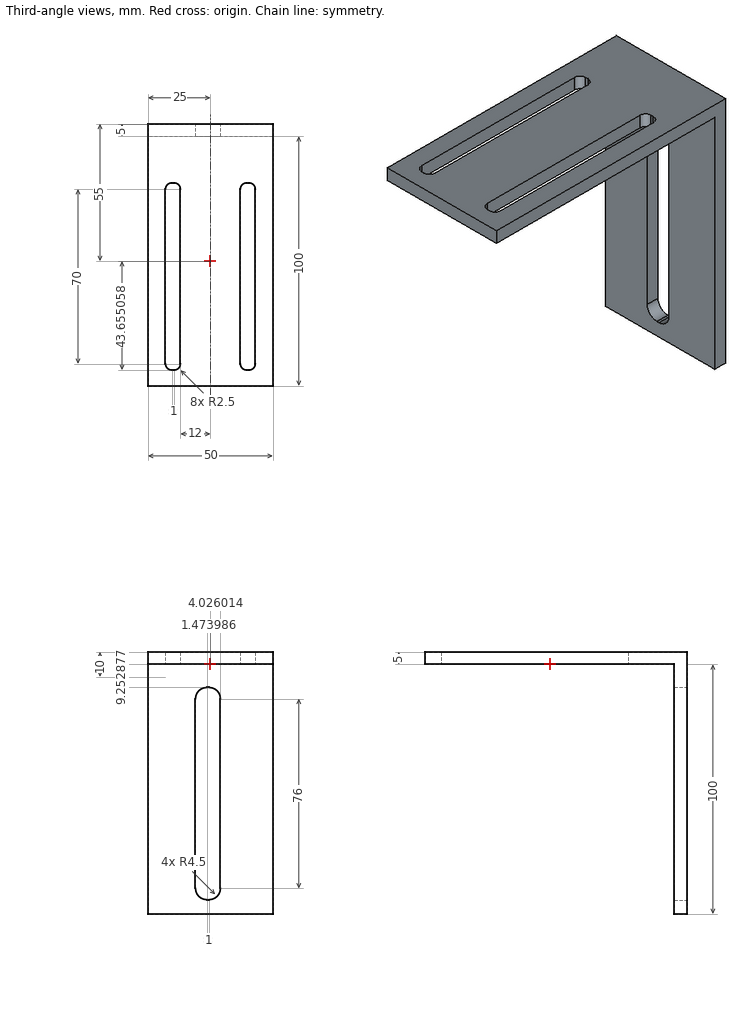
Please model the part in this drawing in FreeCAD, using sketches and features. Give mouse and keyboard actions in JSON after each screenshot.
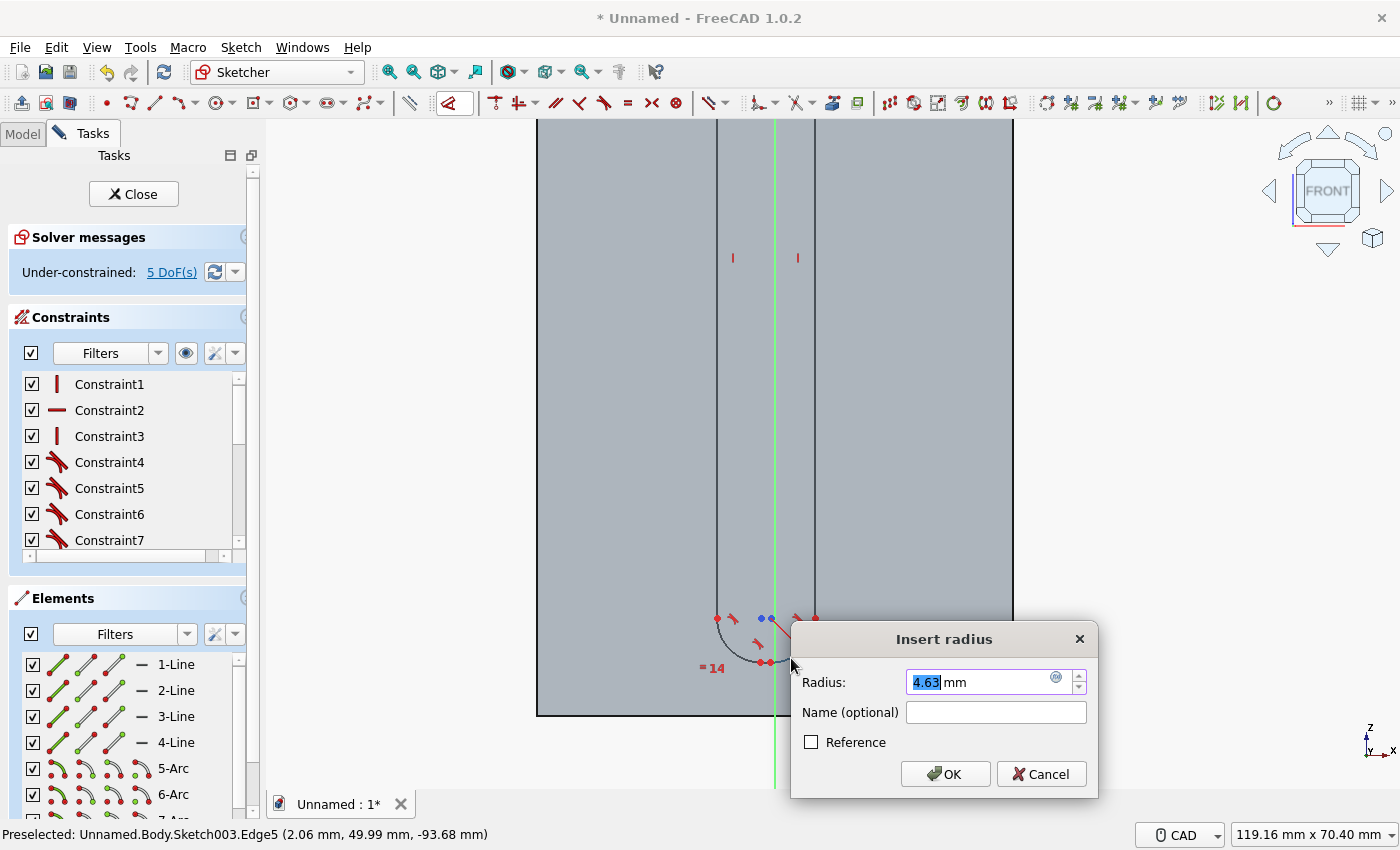
{"action": "type", "text": "4.5"}
{"action": "key", "text": "Return"}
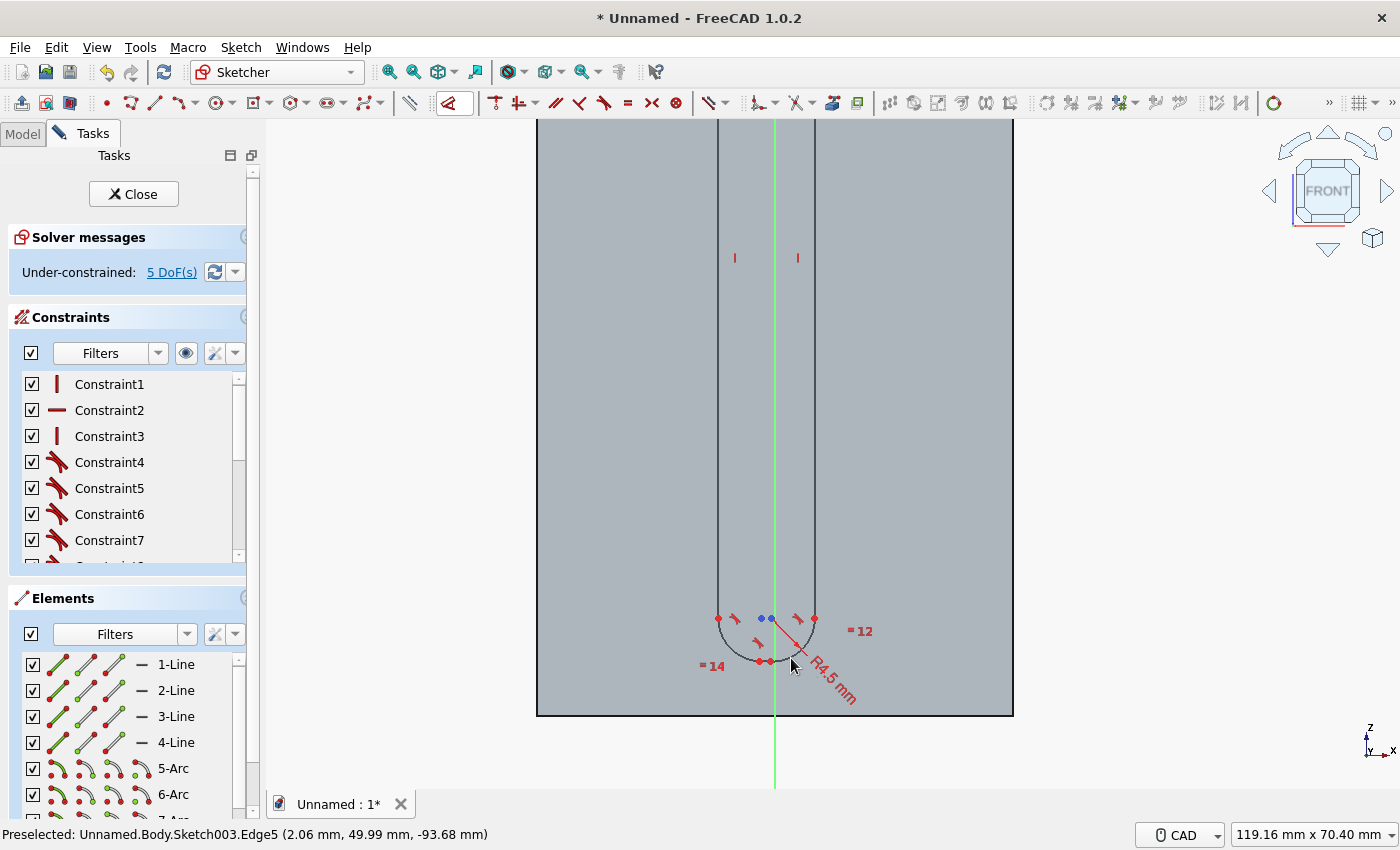
{"action": "scroll", "coordinate": [765, 661], "scroll_direction": "up", "scroll_amount": 8}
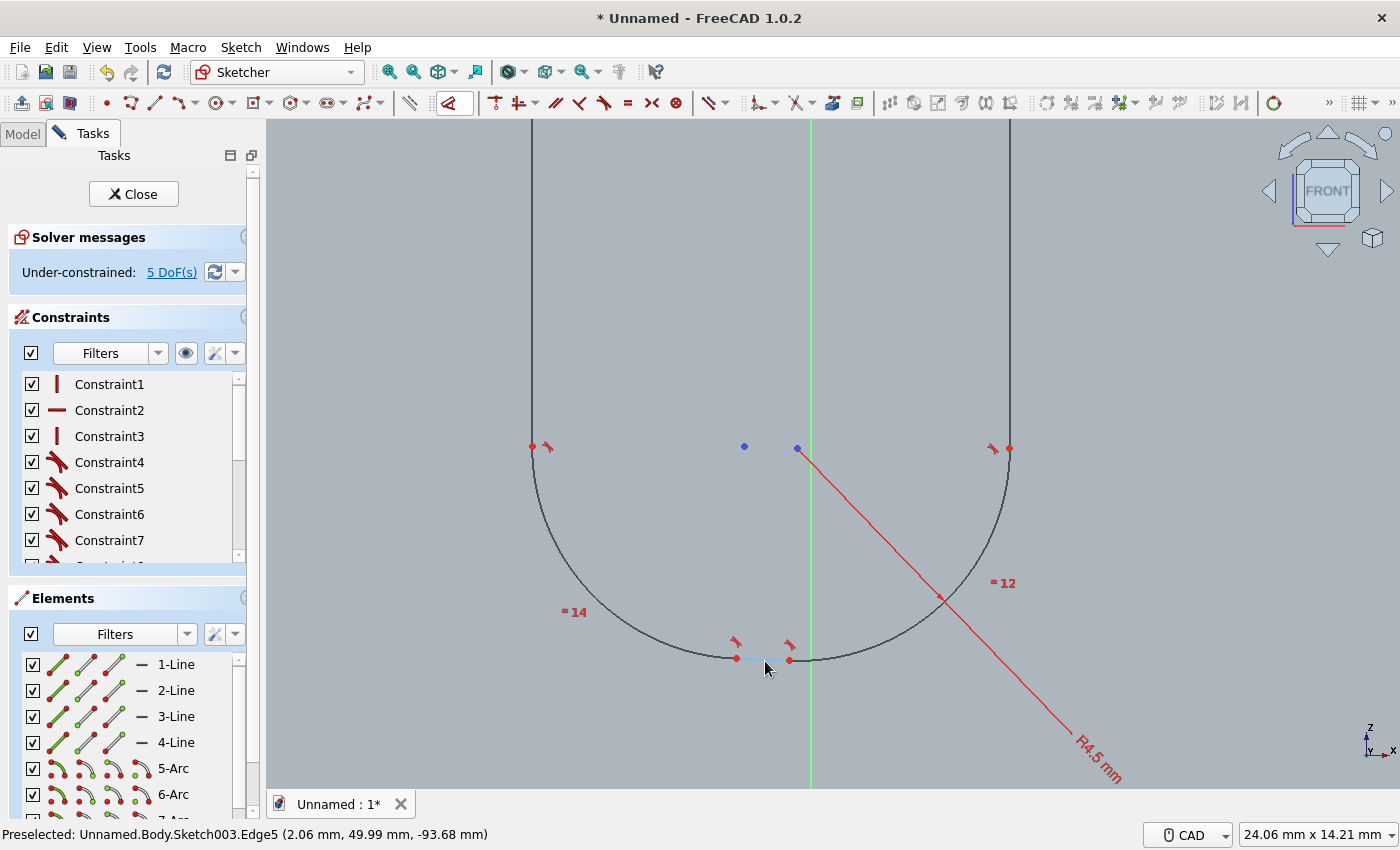
{"action": "left_click", "coordinate": [763, 660]}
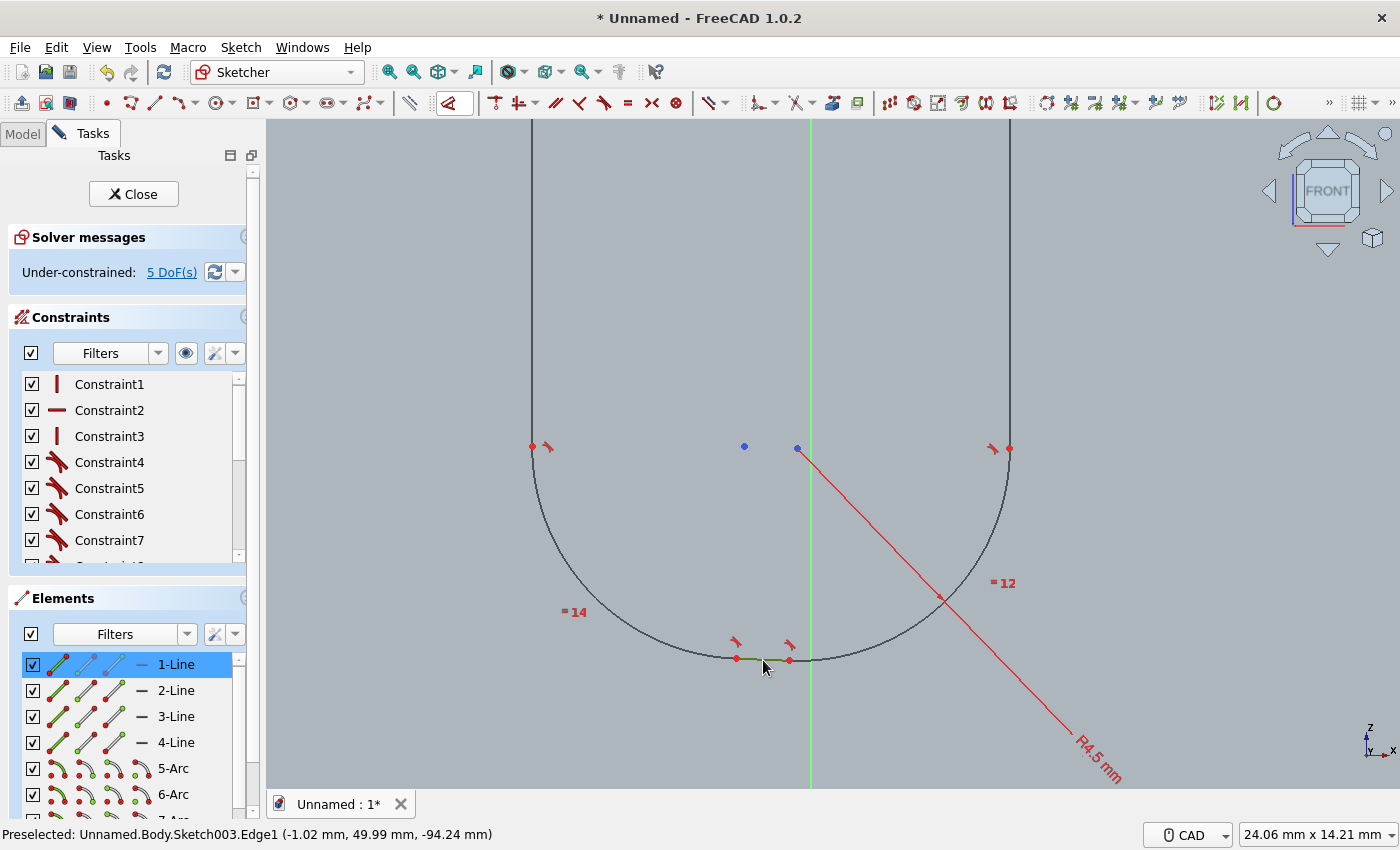
{"action": "left_click", "coordinate": [468, 104]}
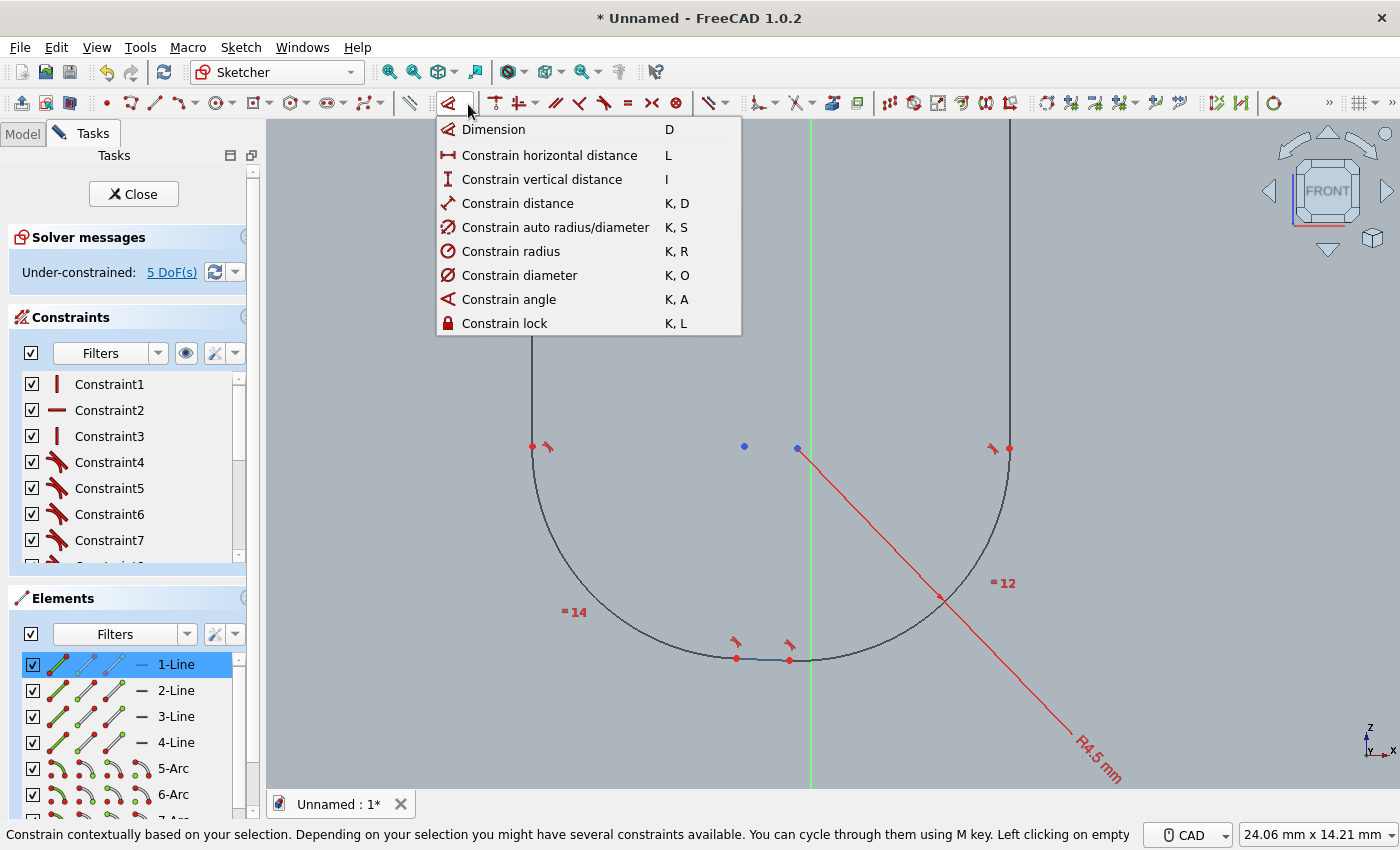
{"action": "left_click", "coordinate": [589, 155]}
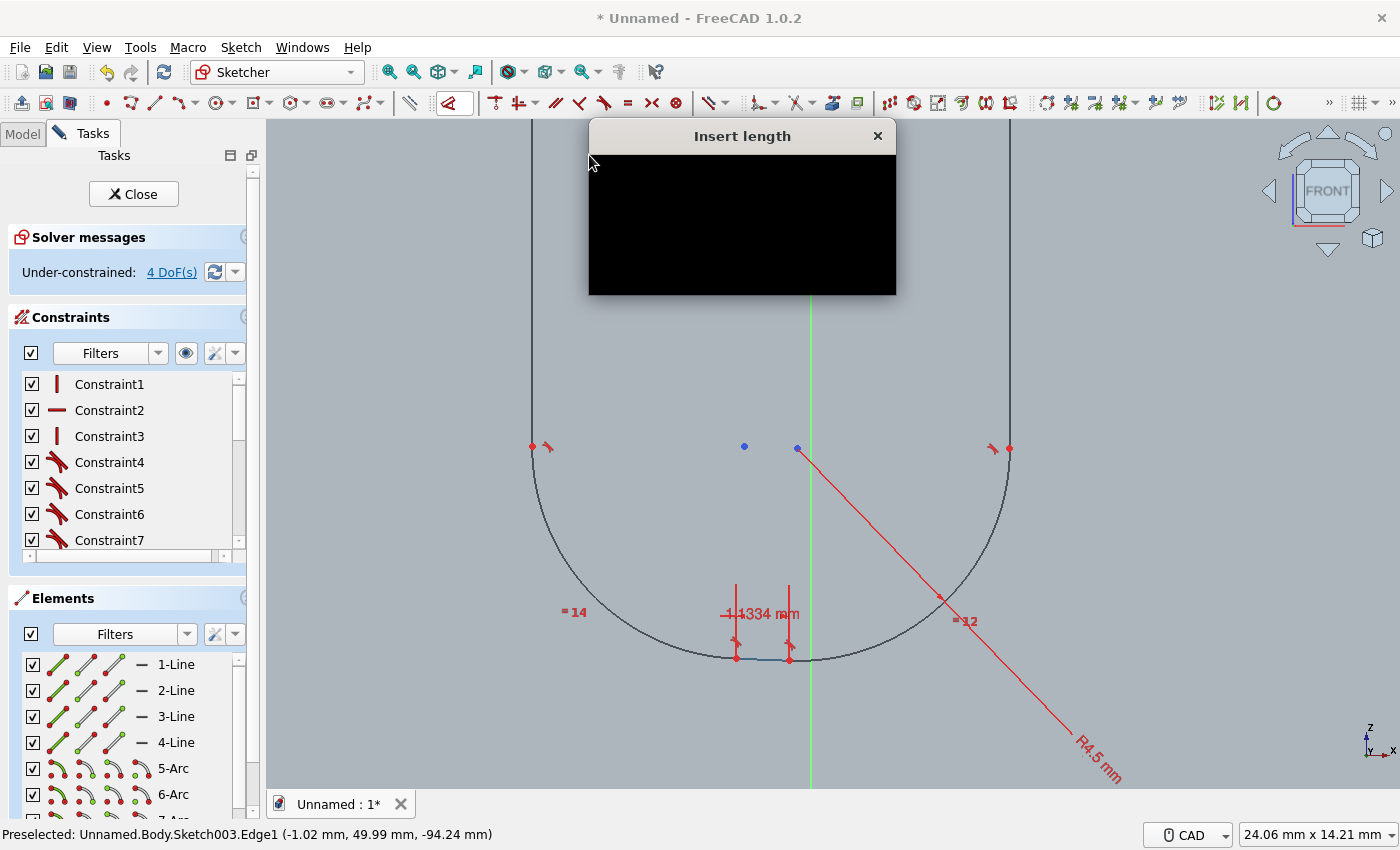
{"action": "type", "text": "1"}
{"action": "key", "text": "Return"}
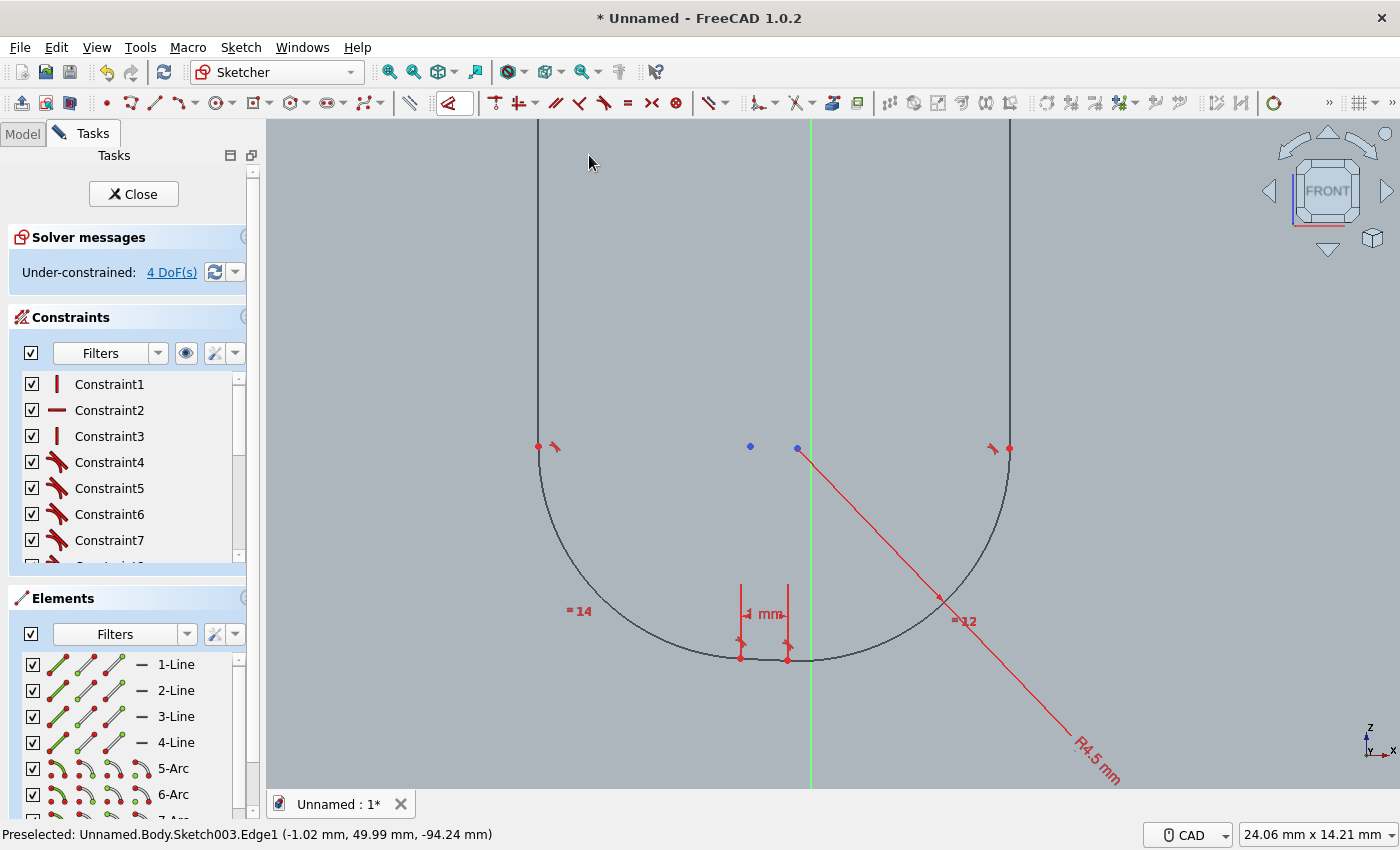
{"action": "scroll", "coordinate": [764, 655], "scroll_direction": "down", "scroll_amount": 12}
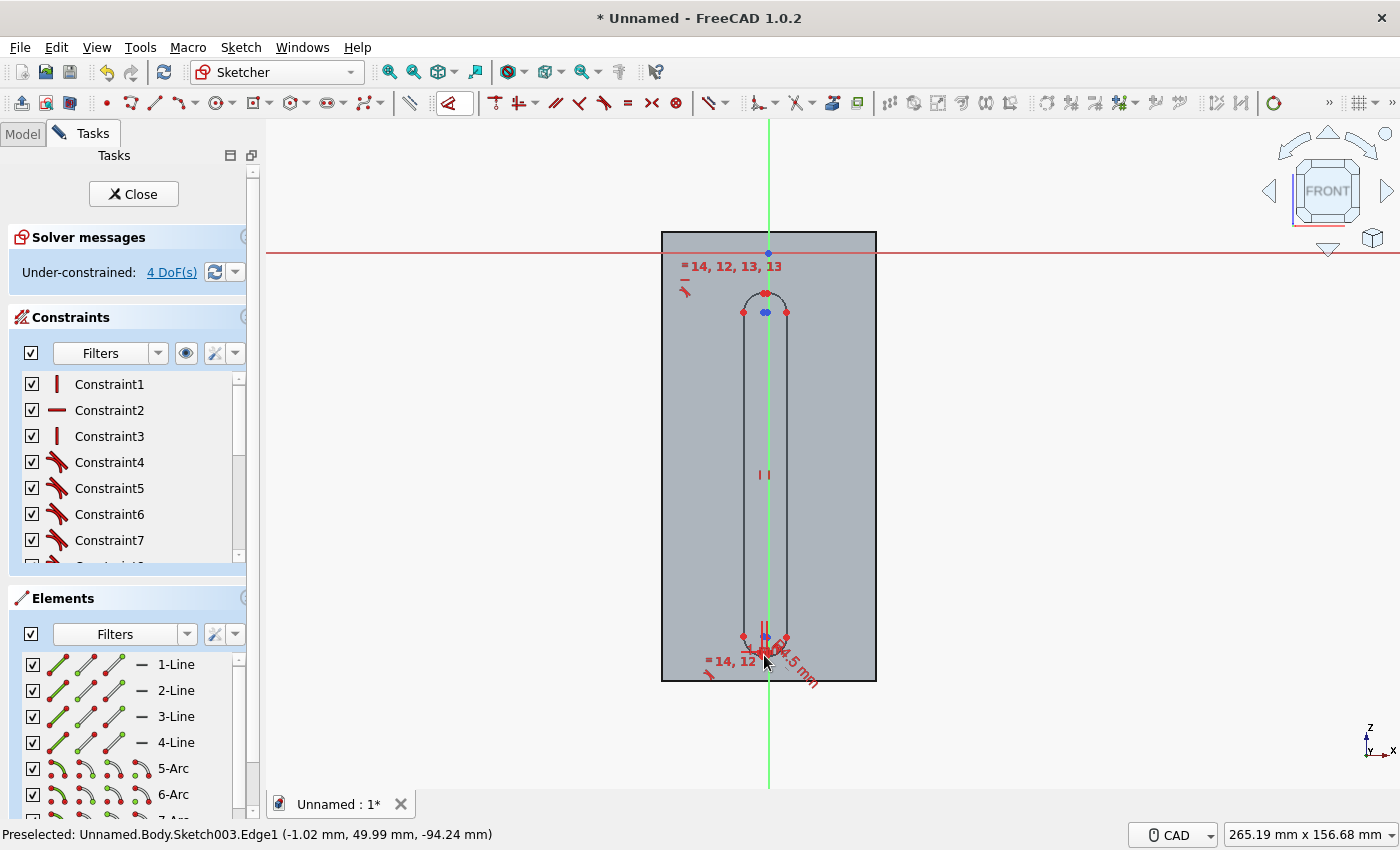
{"action": "left_click", "coordinate": [787, 540]}